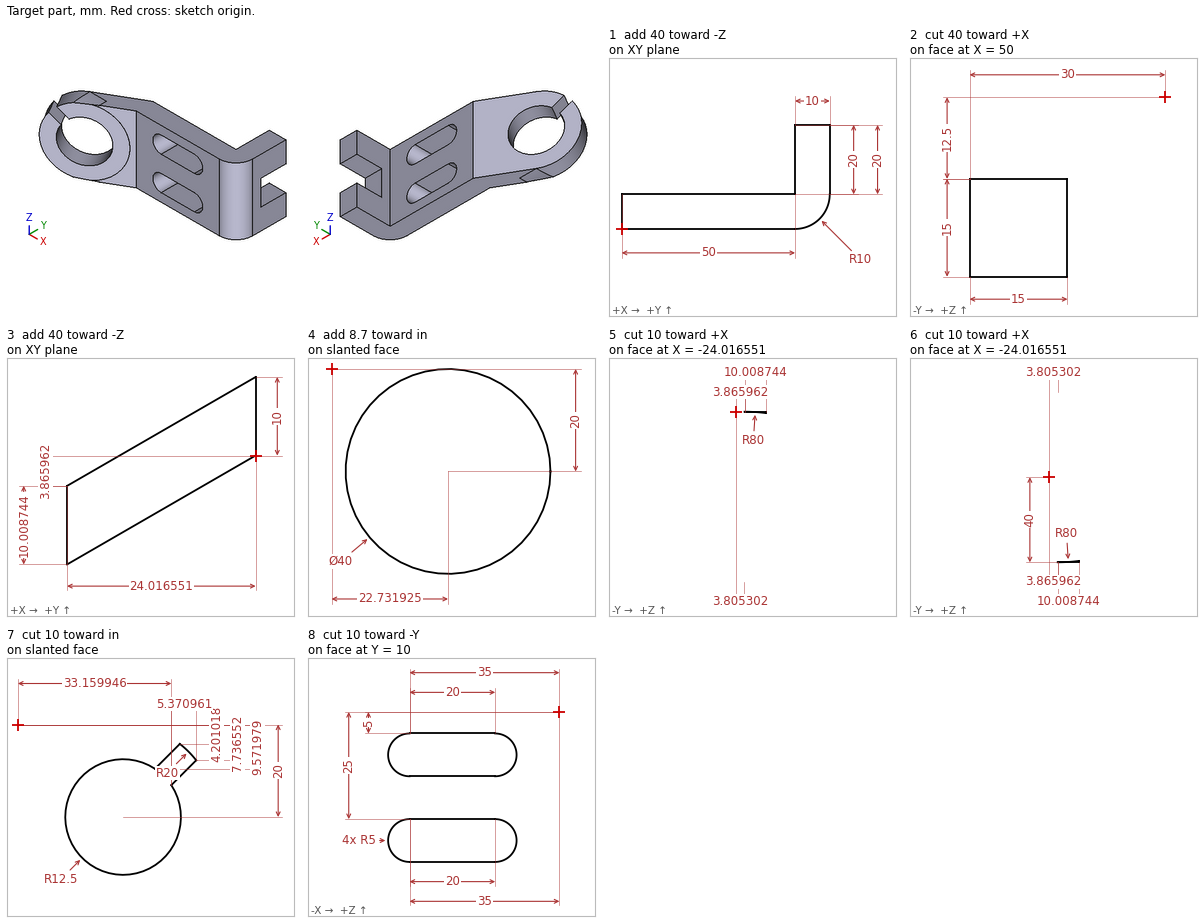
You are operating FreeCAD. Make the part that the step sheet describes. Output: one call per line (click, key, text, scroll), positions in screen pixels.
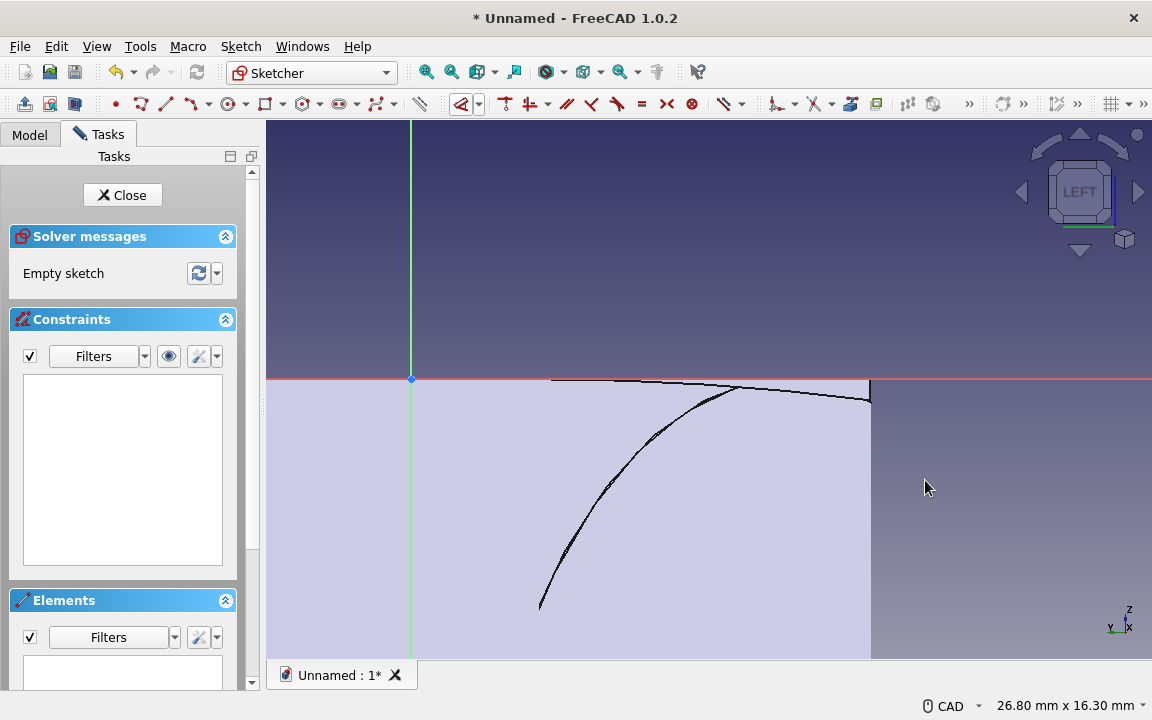
click(141, 104)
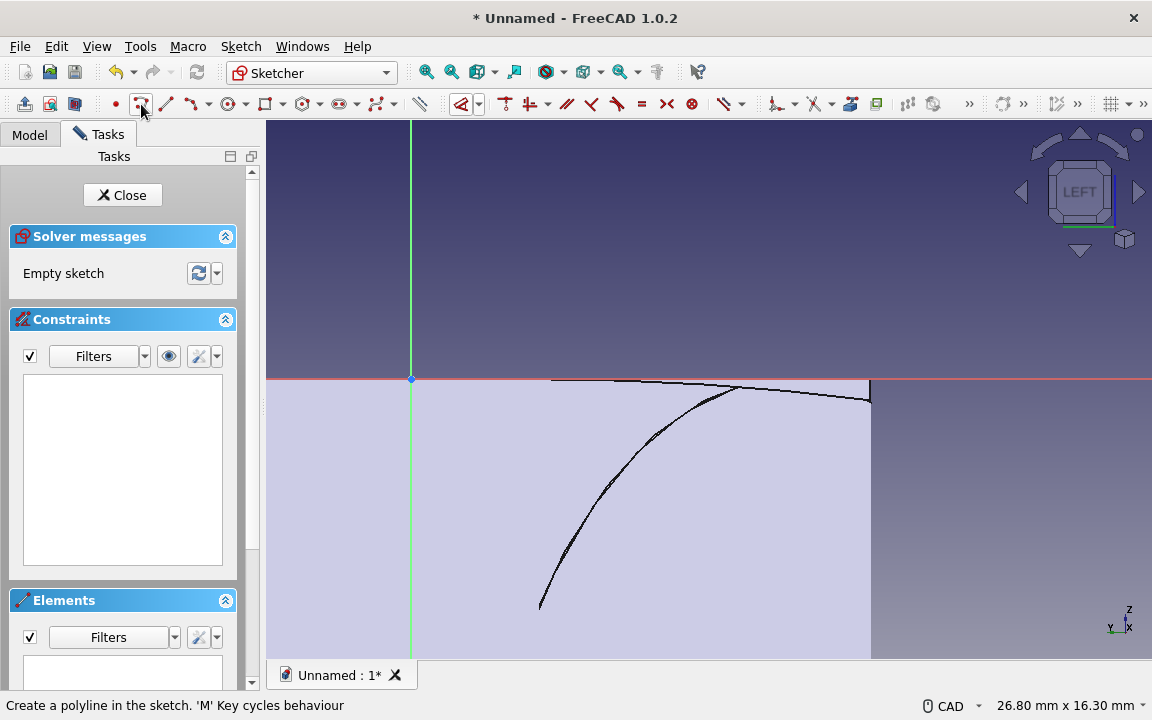
click(870, 400)
click(870, 379)
click(539, 388)
right_click(539, 388)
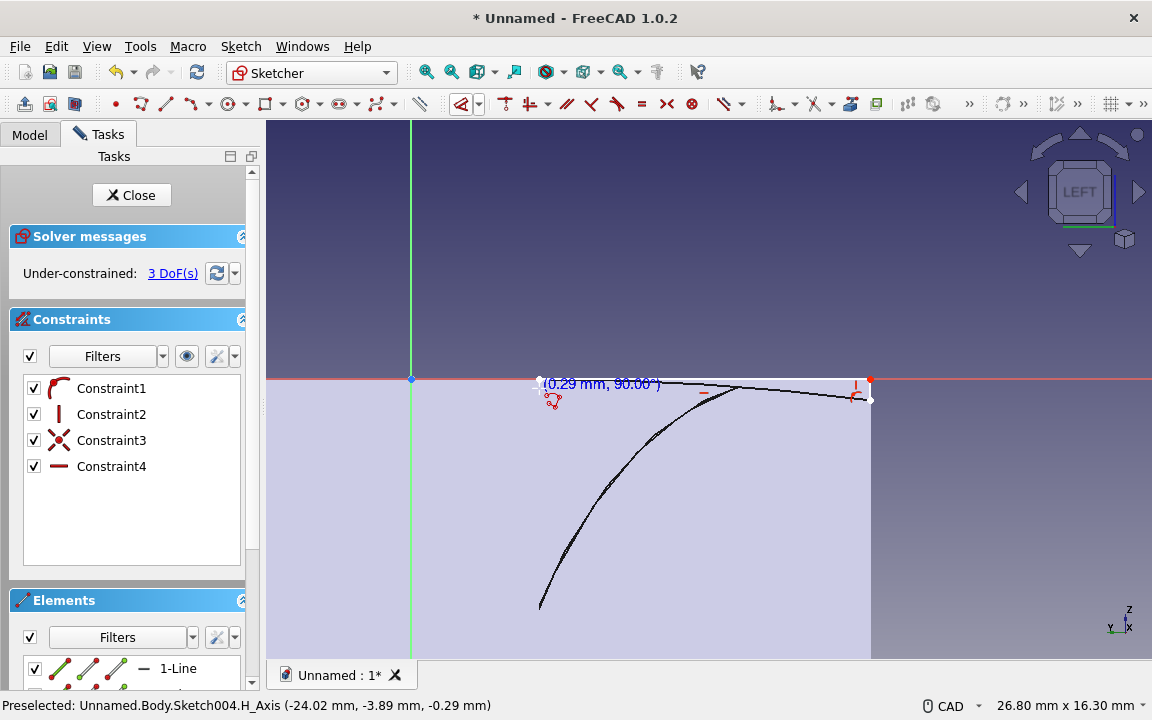
click(190, 104)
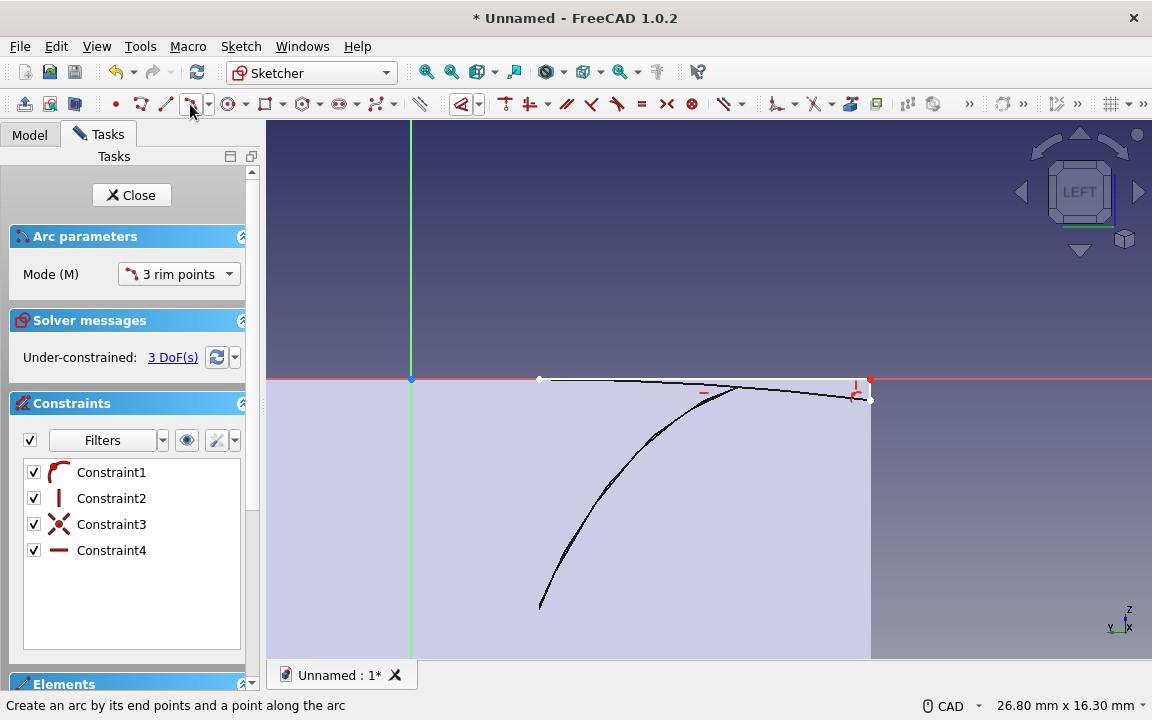
click(539, 379)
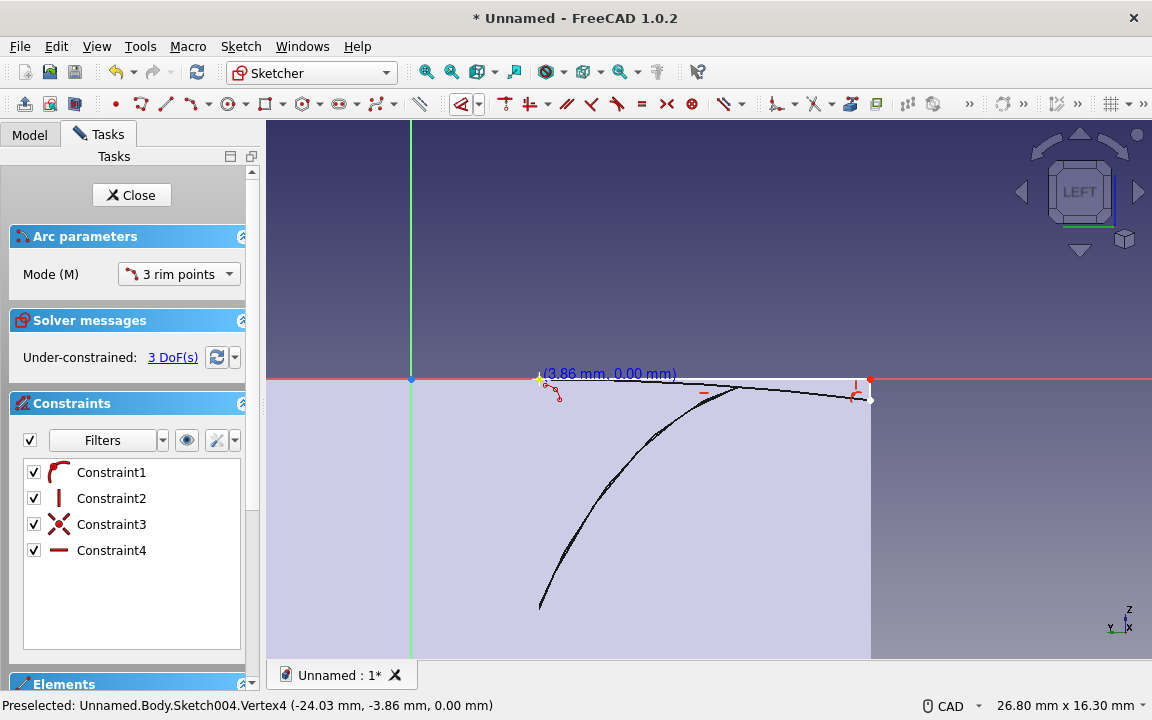
scroll(870, 400, up, 3)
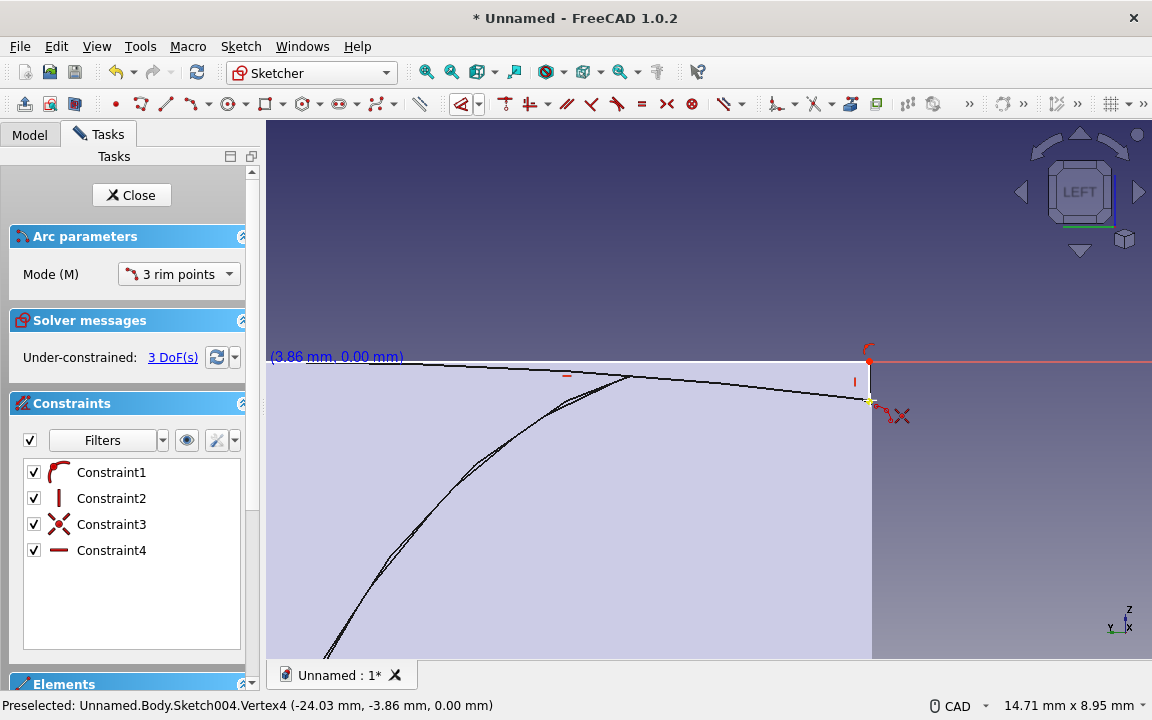
click(869, 401)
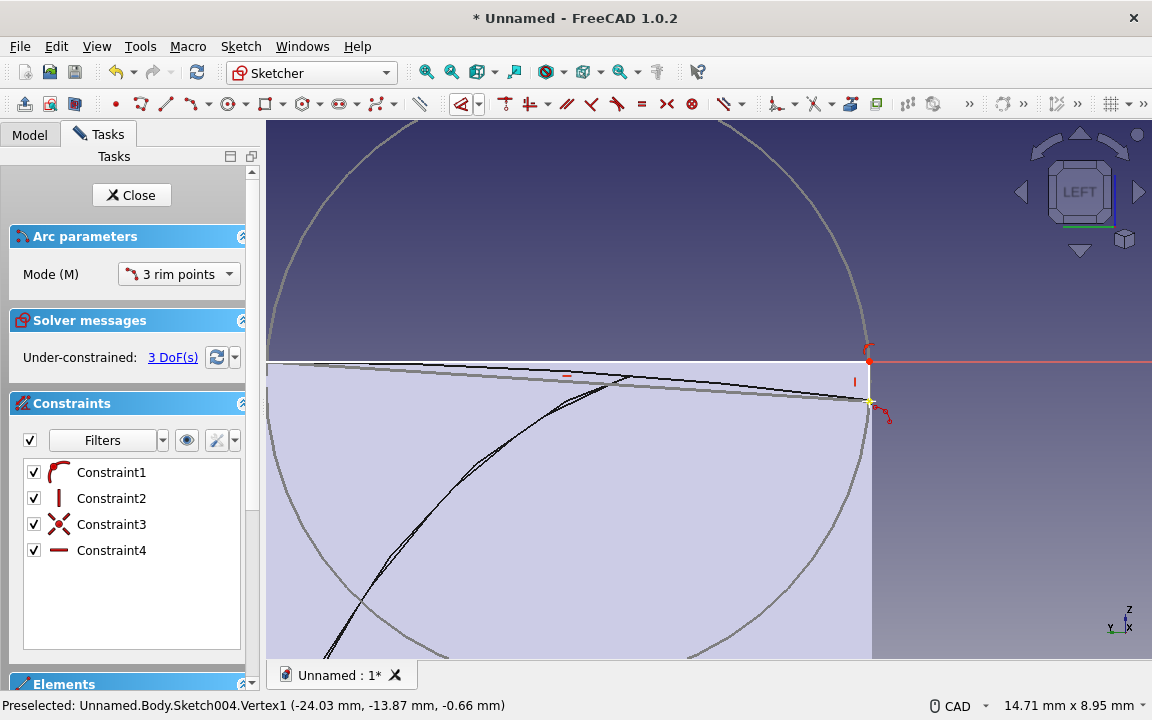
scroll(569, 372, up, 3)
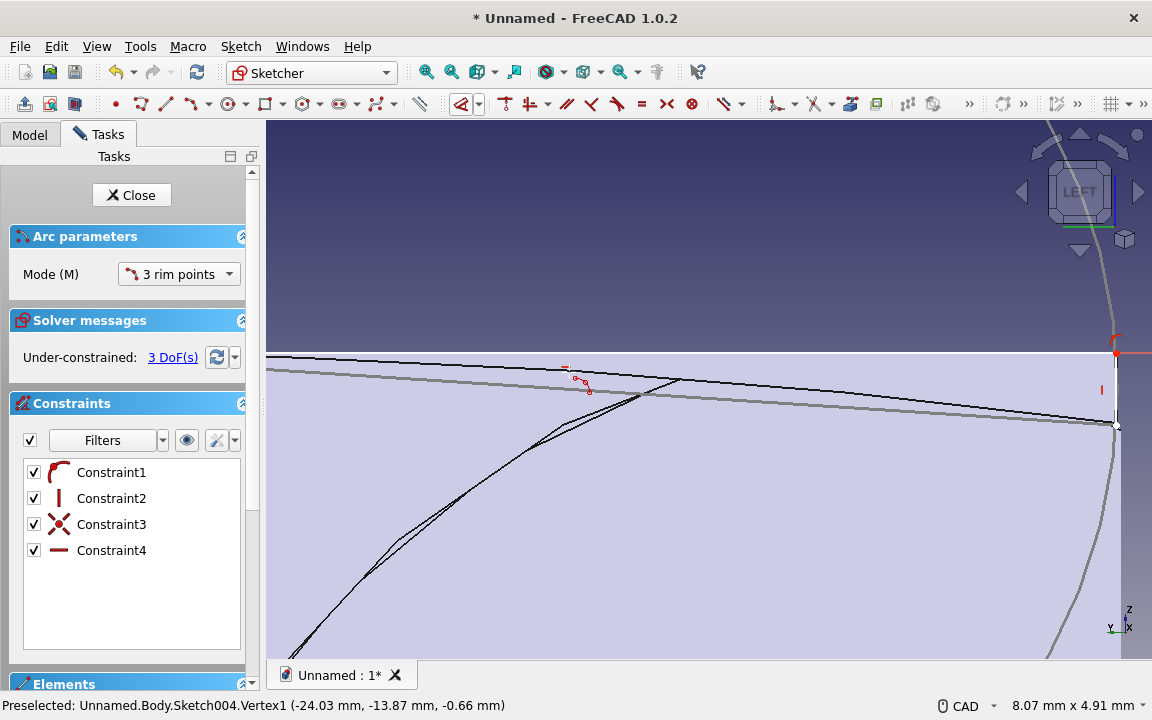
click(568, 371)
key(Escape)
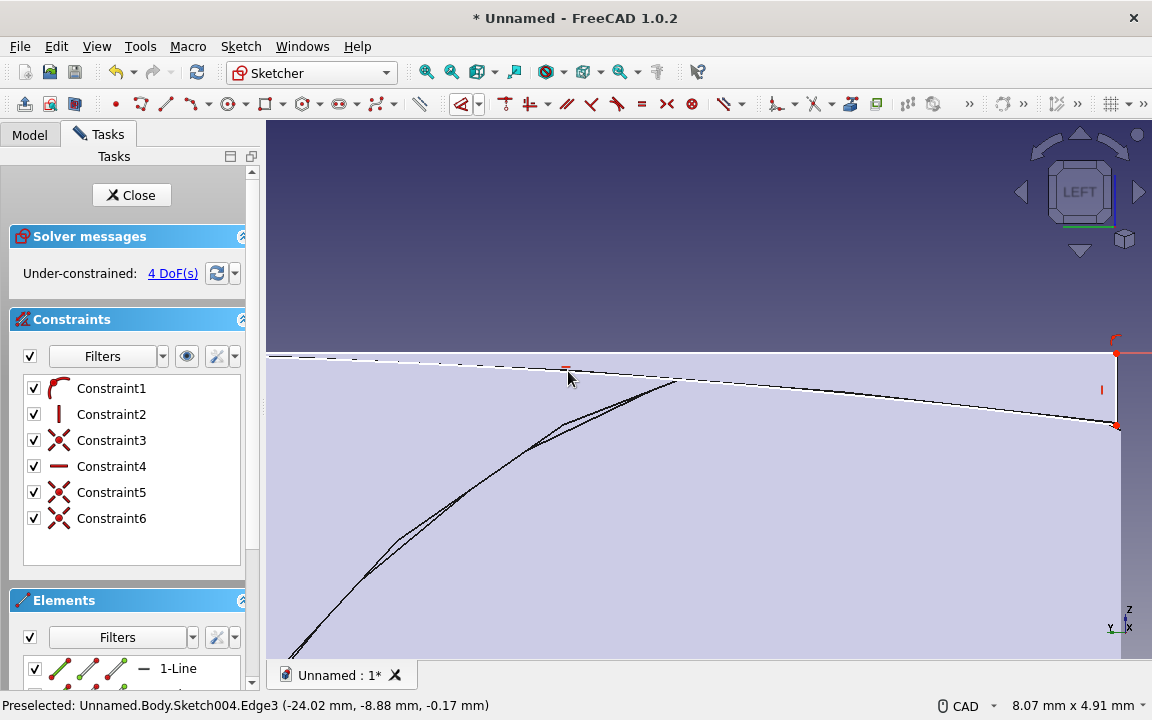
click(788, 389)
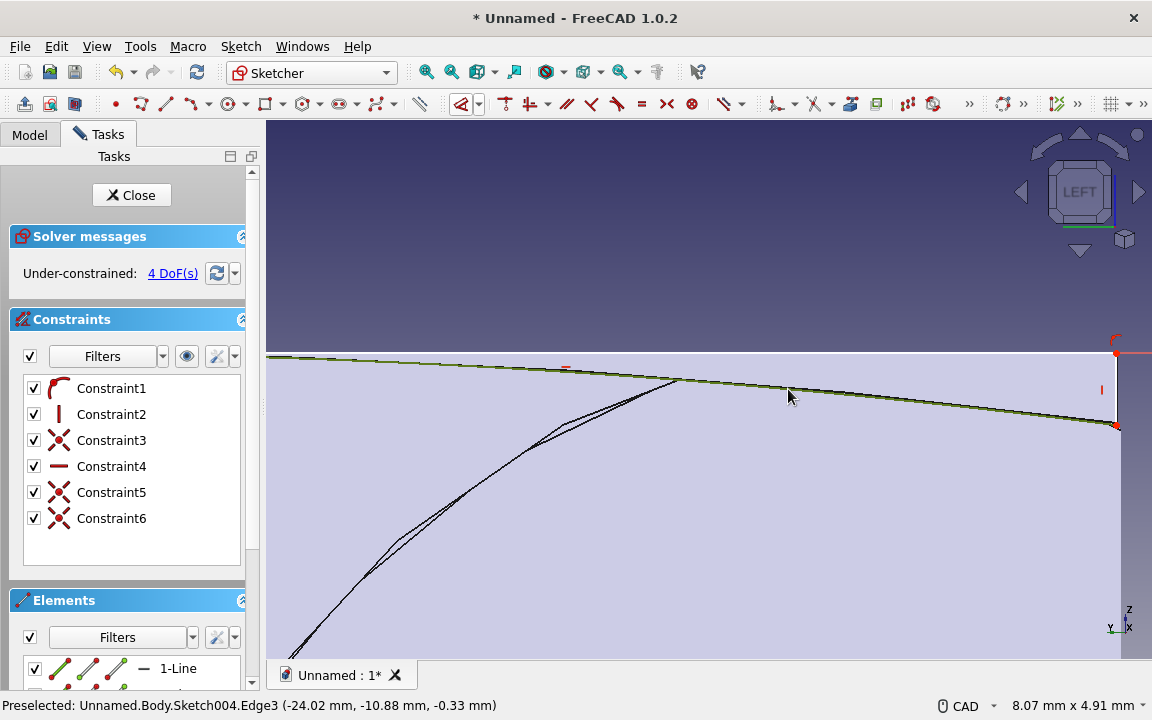
key(k)
key(r)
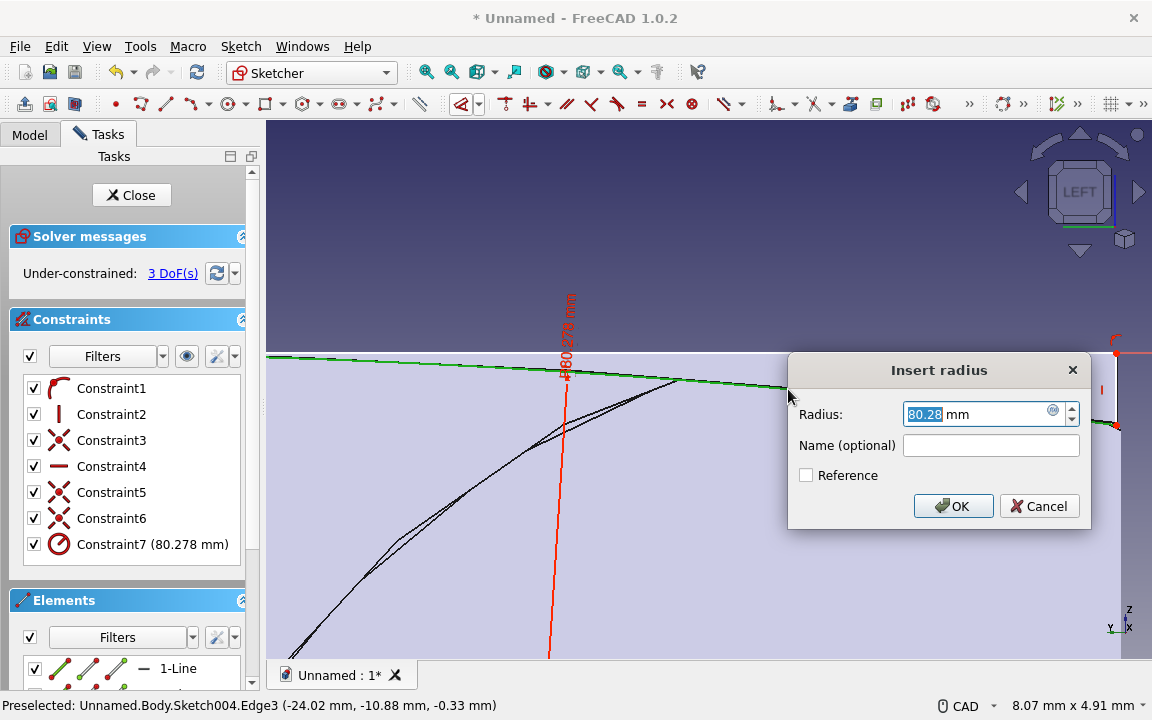
text(80)
key(Return)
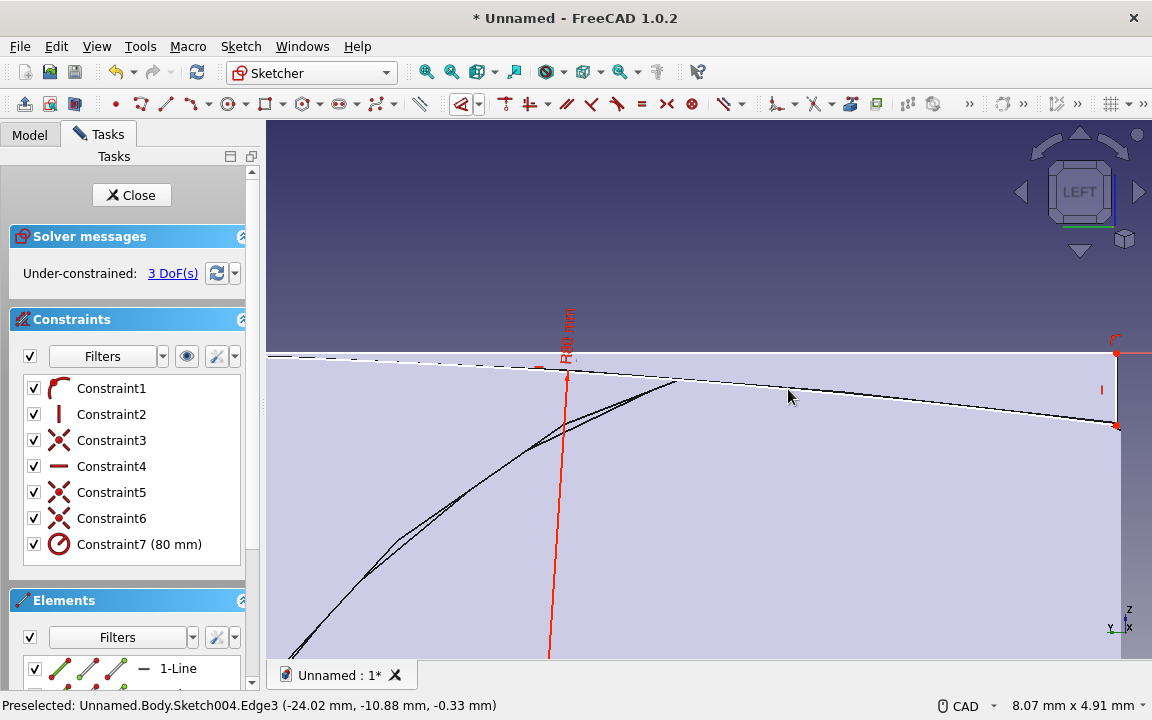
click(786, 353)